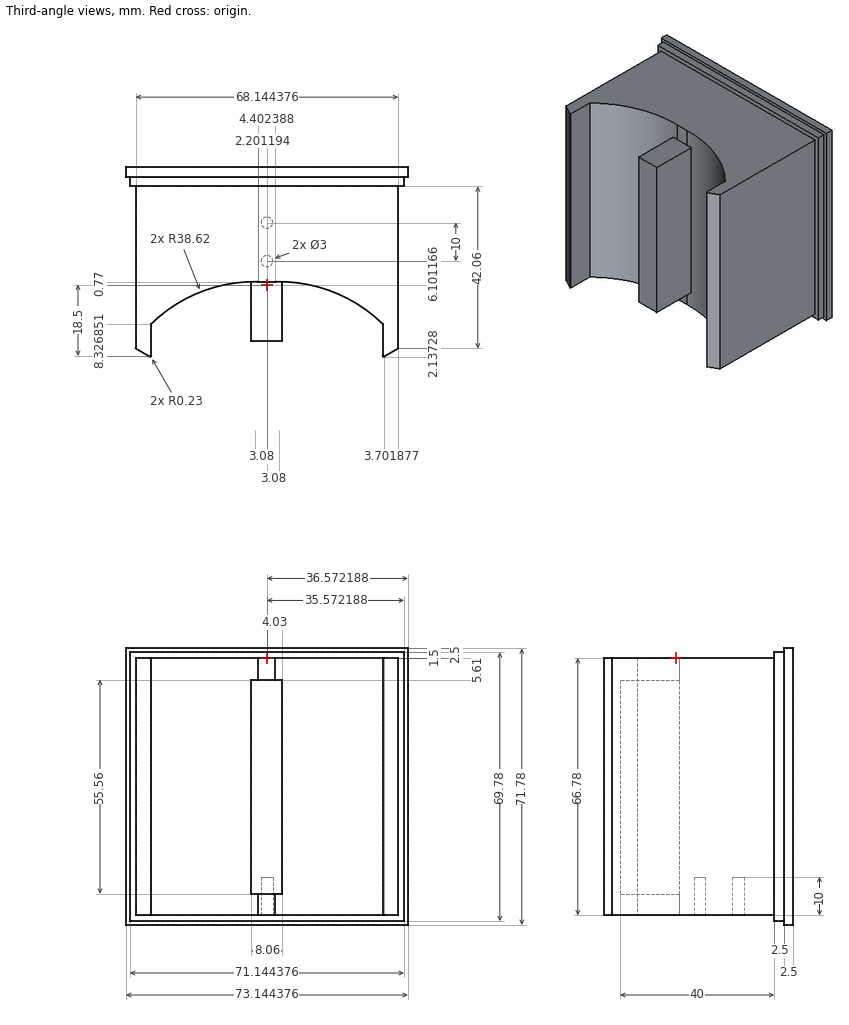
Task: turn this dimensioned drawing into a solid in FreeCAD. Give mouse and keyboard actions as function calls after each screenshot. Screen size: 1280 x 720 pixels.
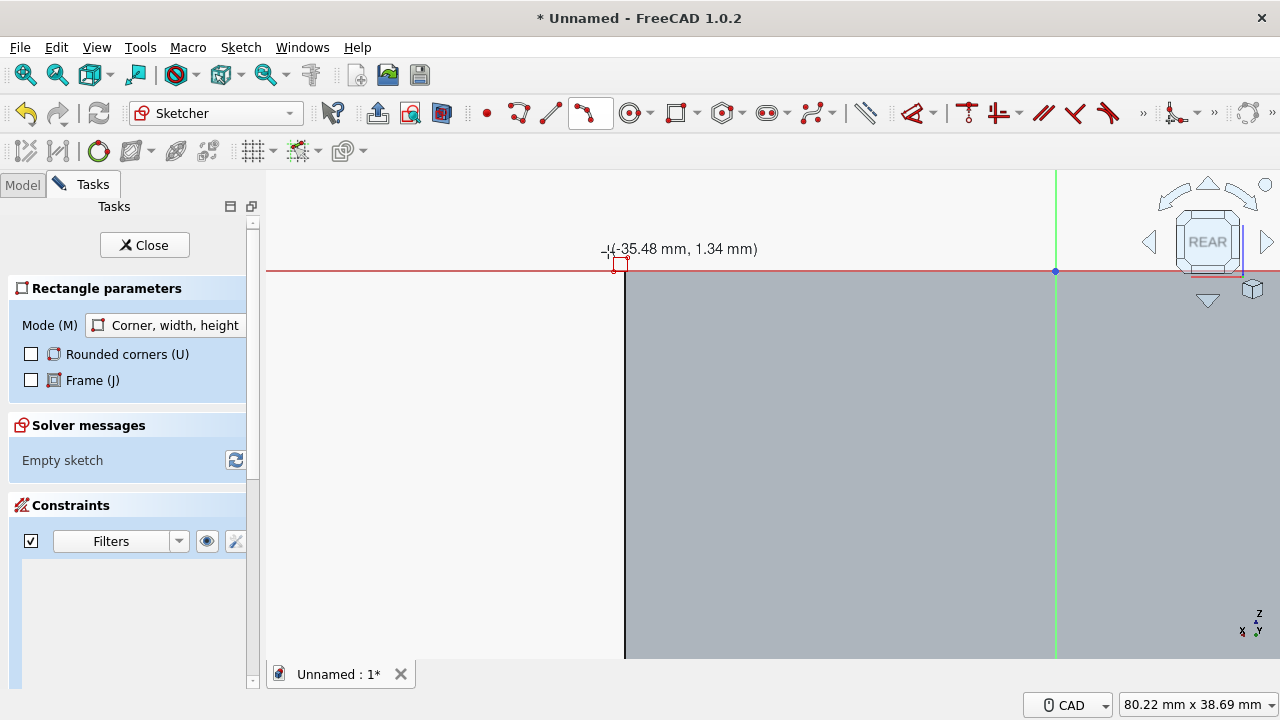
click(606, 252)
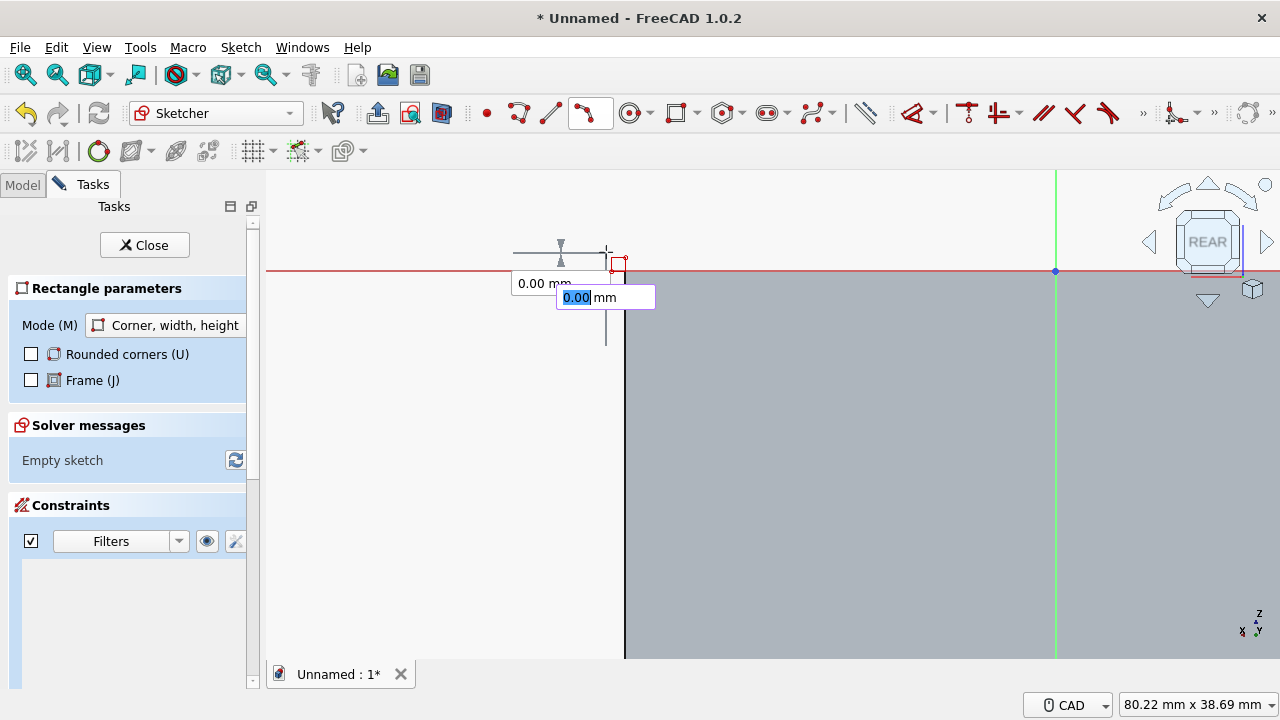
scroll(500, 252, down, 5)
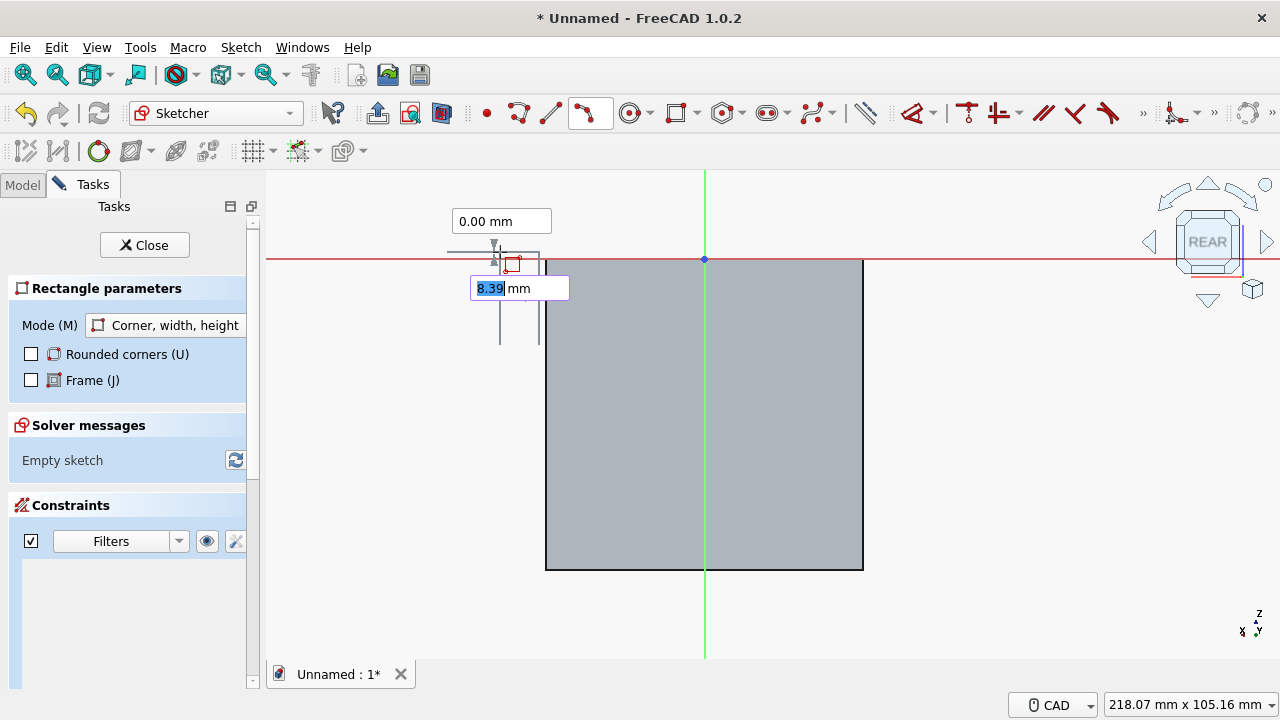
click(870, 577)
key(Escape)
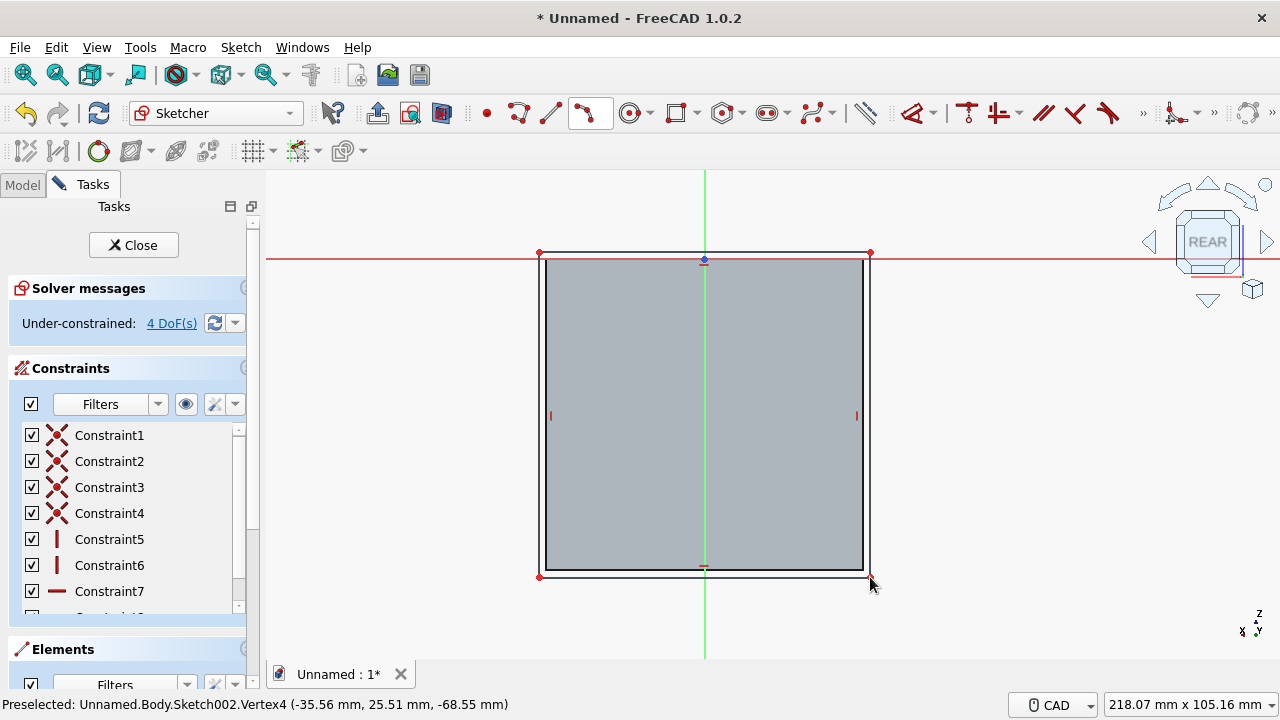
click(912, 114)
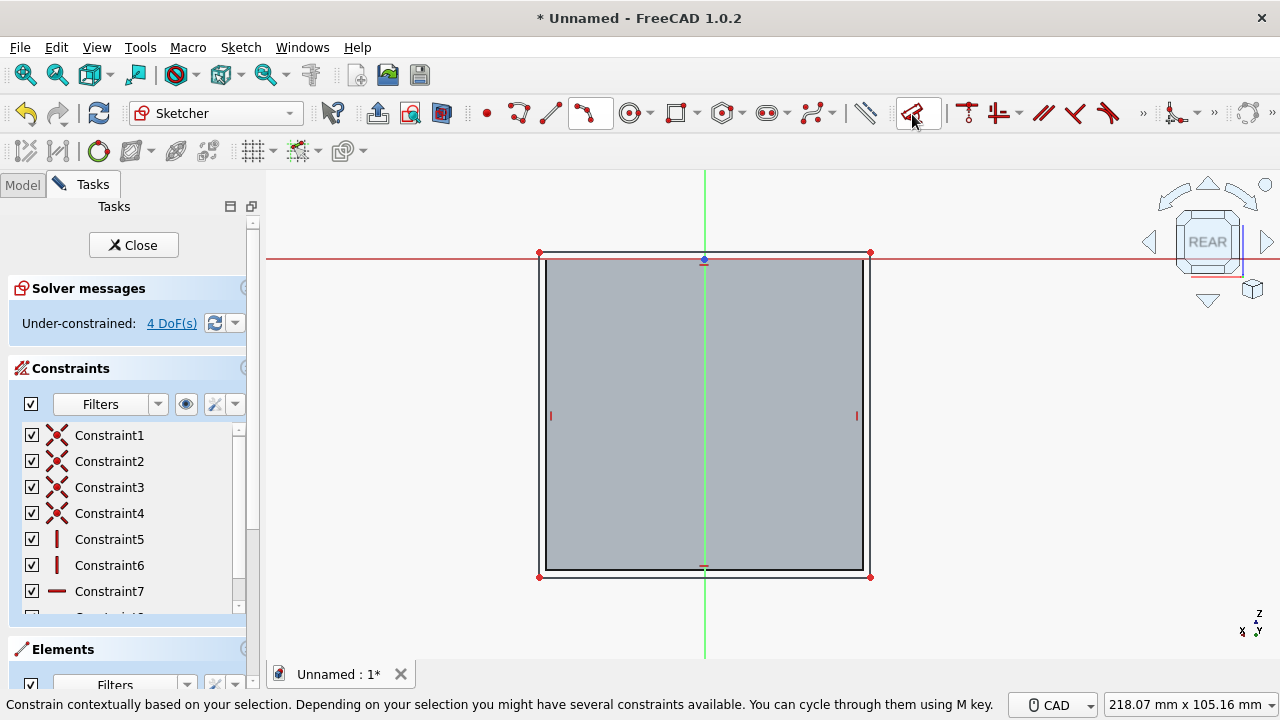
scroll(539, 252, up, 9)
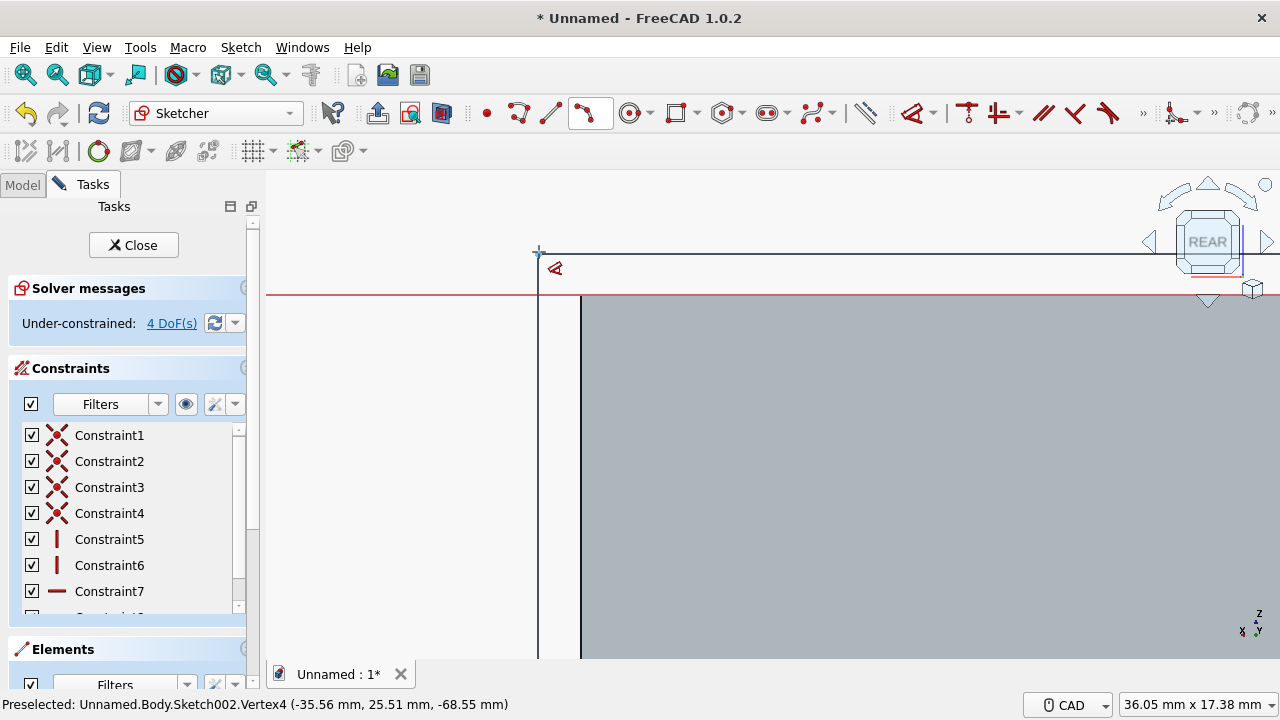
click(538, 254)
click(504, 274)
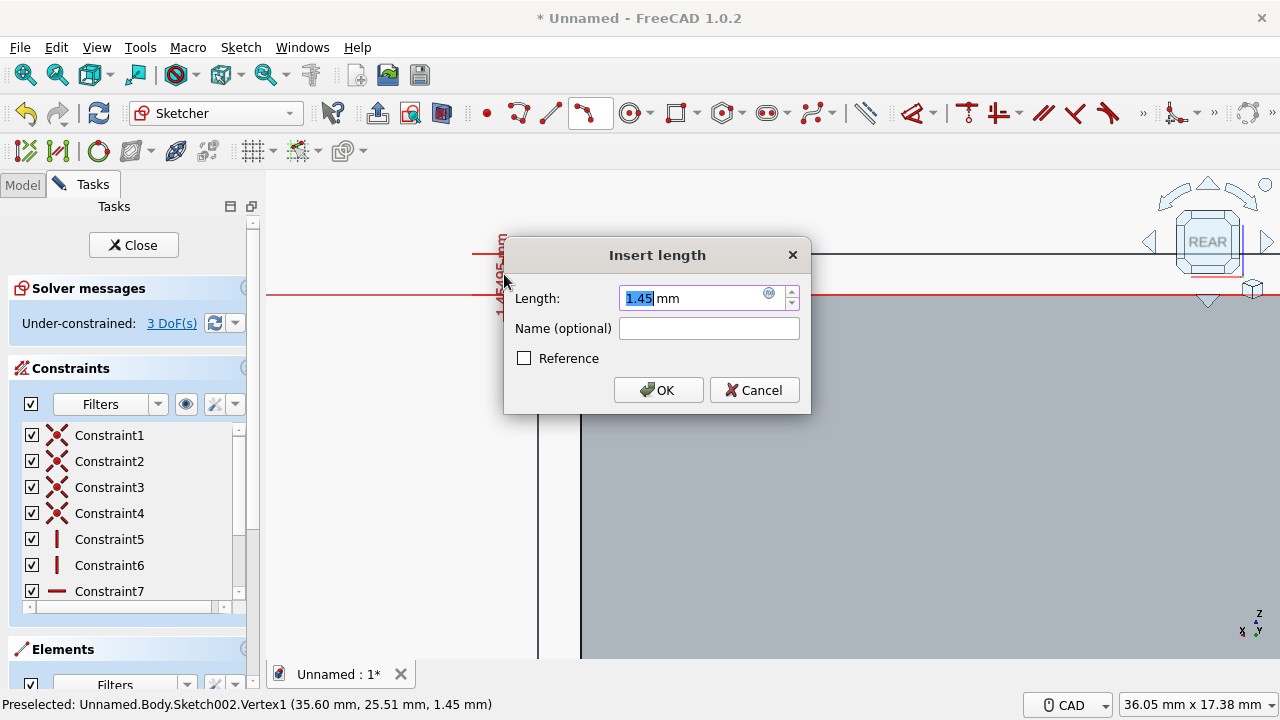
text(1.5)
key(Return)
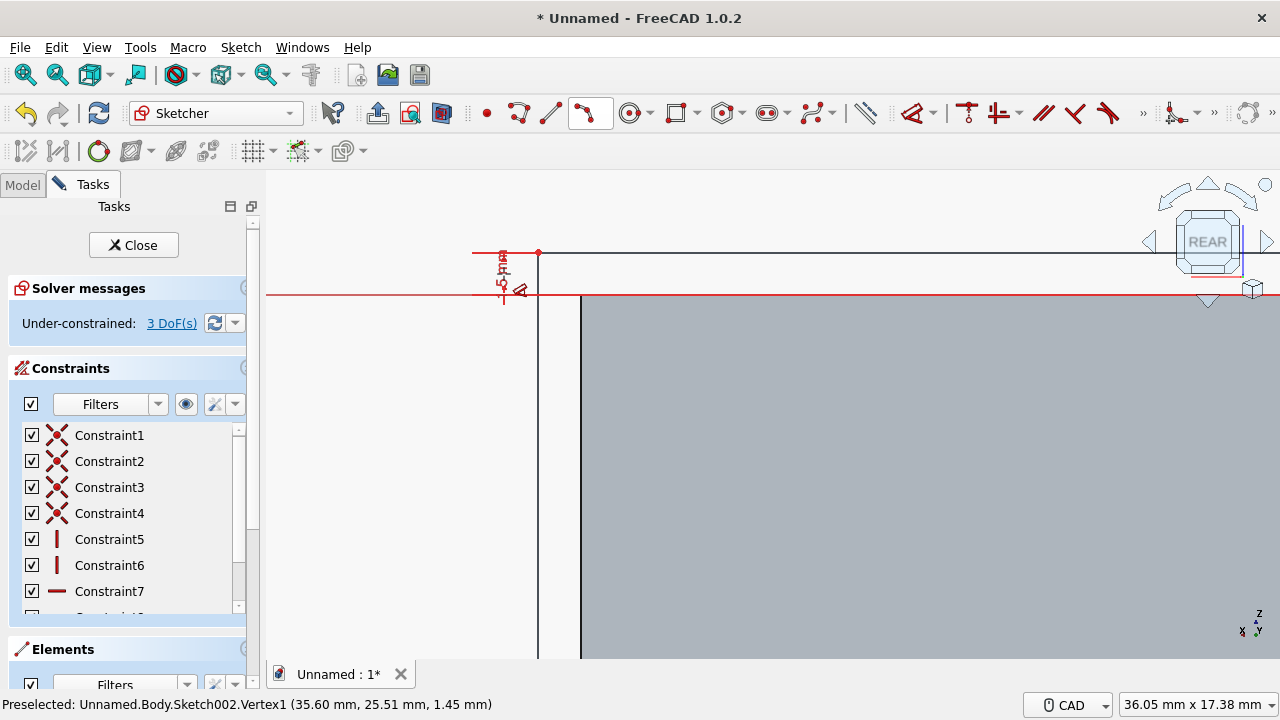
scroll(539, 252, down, 9)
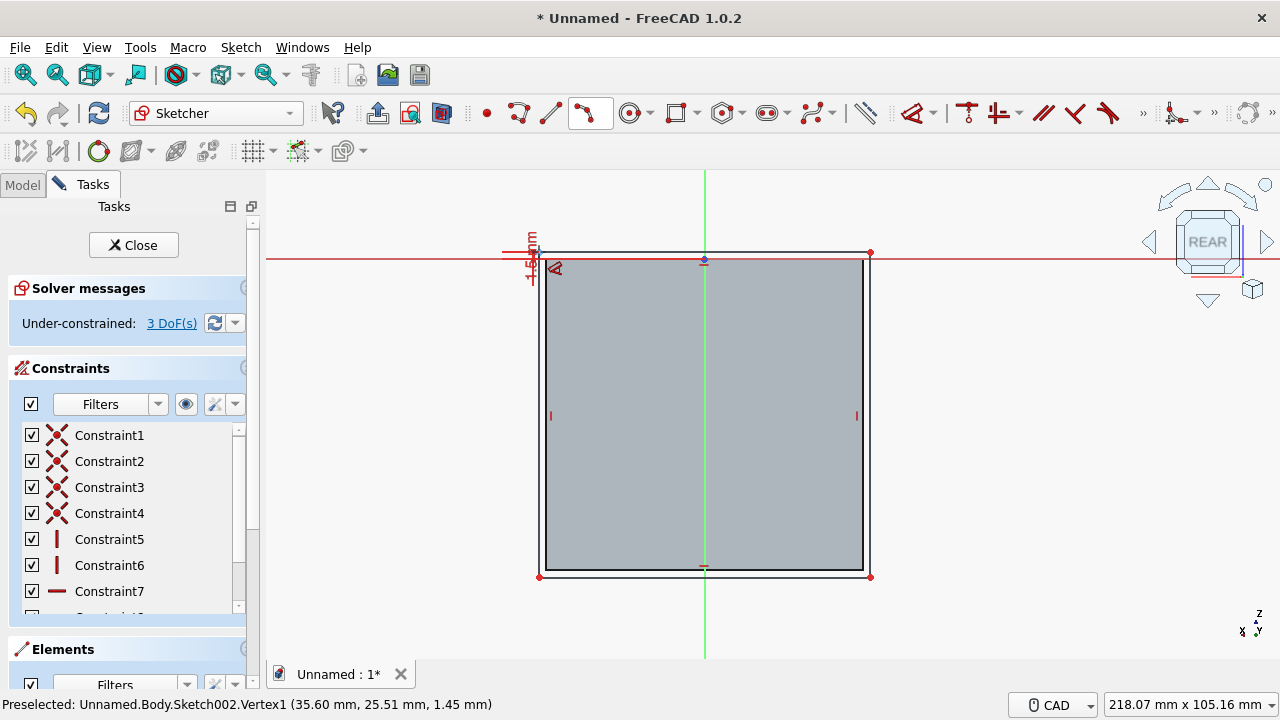
click(539, 350)
click(505, 415)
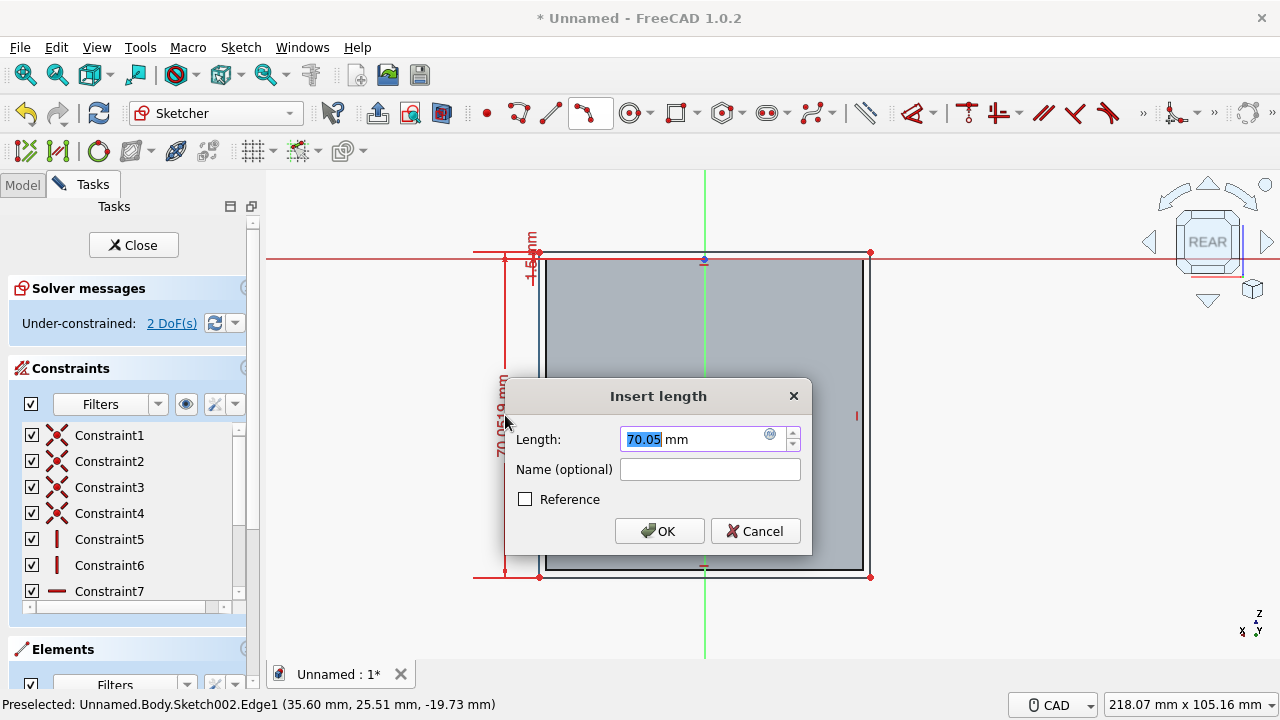
text(69.78)
key(Return)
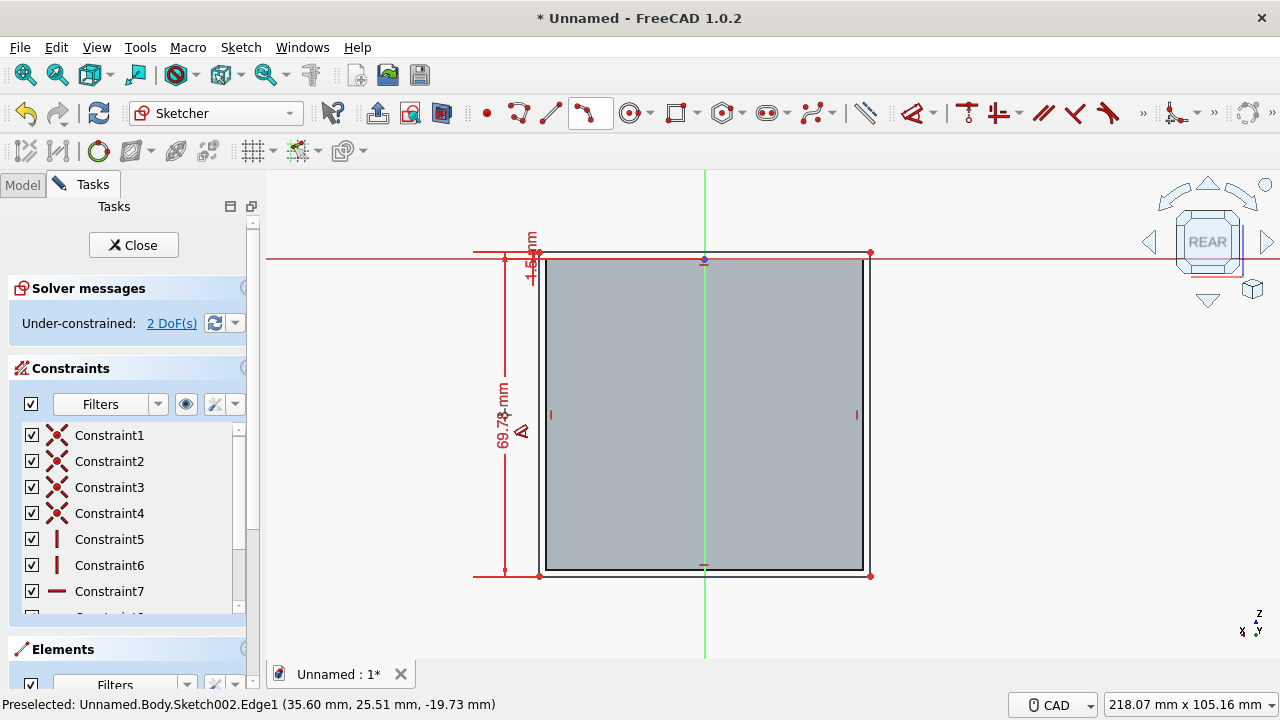
click(638, 577)
click(628, 611)